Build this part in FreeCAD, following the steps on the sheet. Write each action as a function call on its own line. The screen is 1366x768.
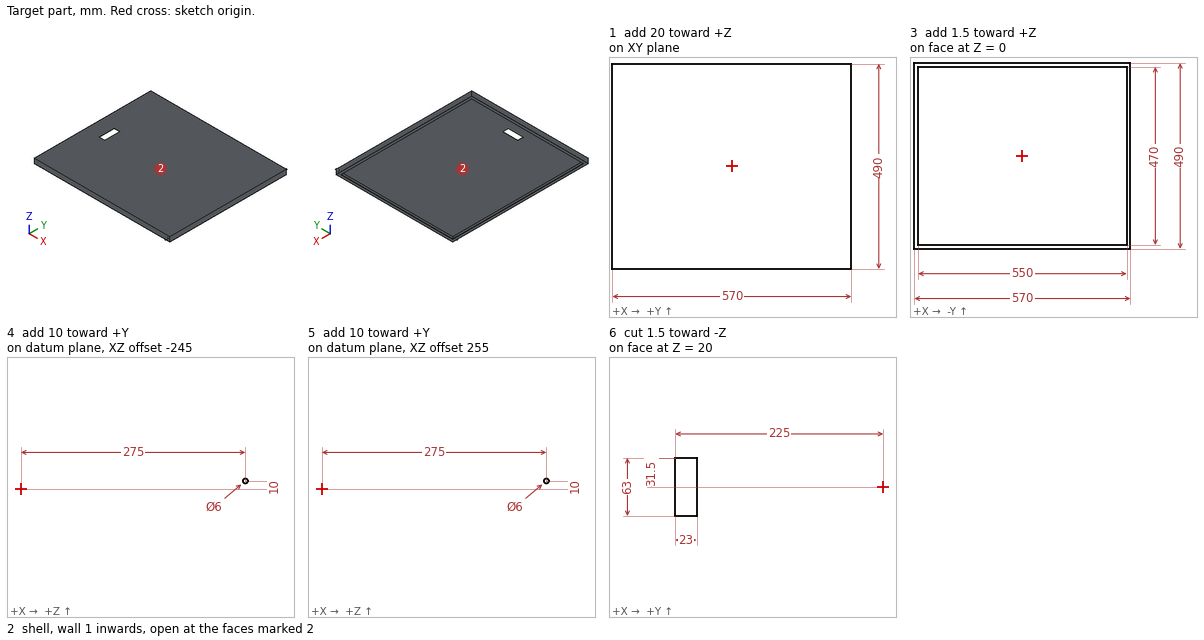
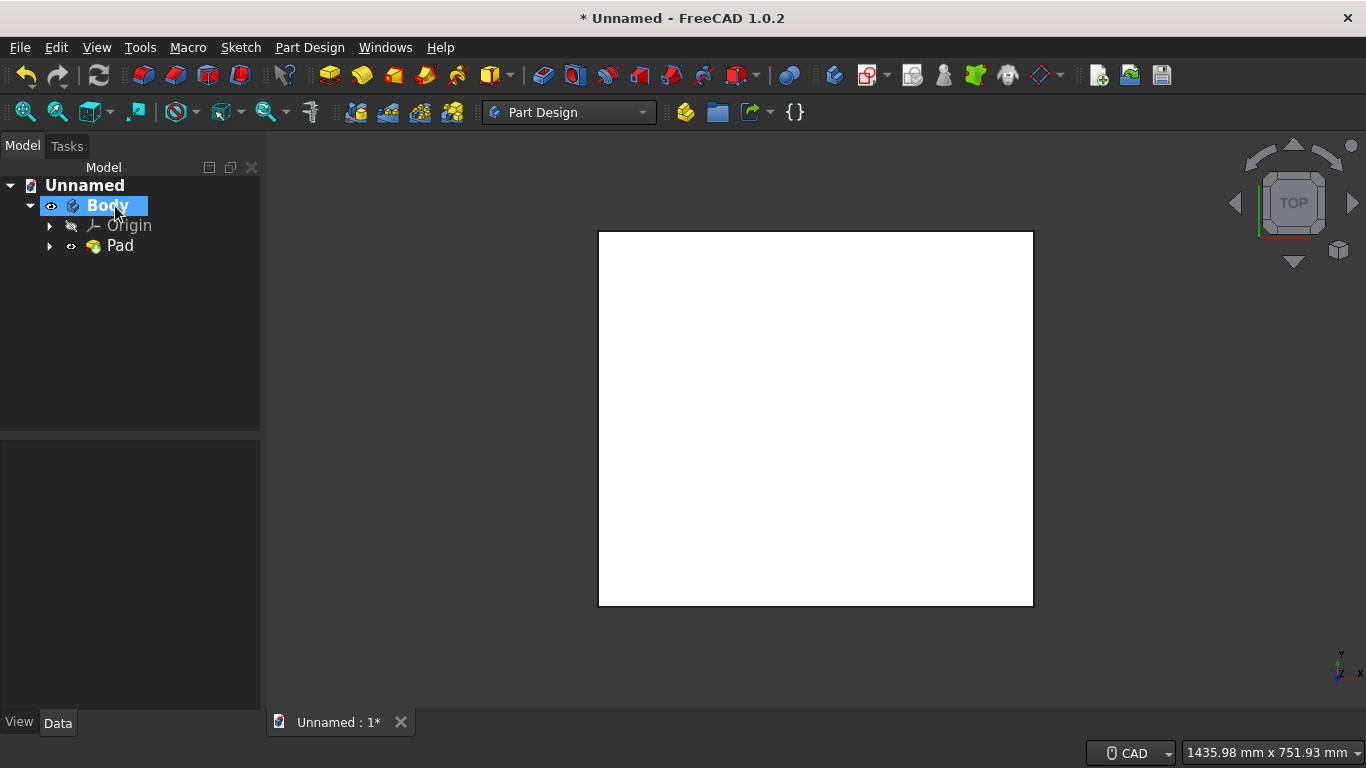
key(1)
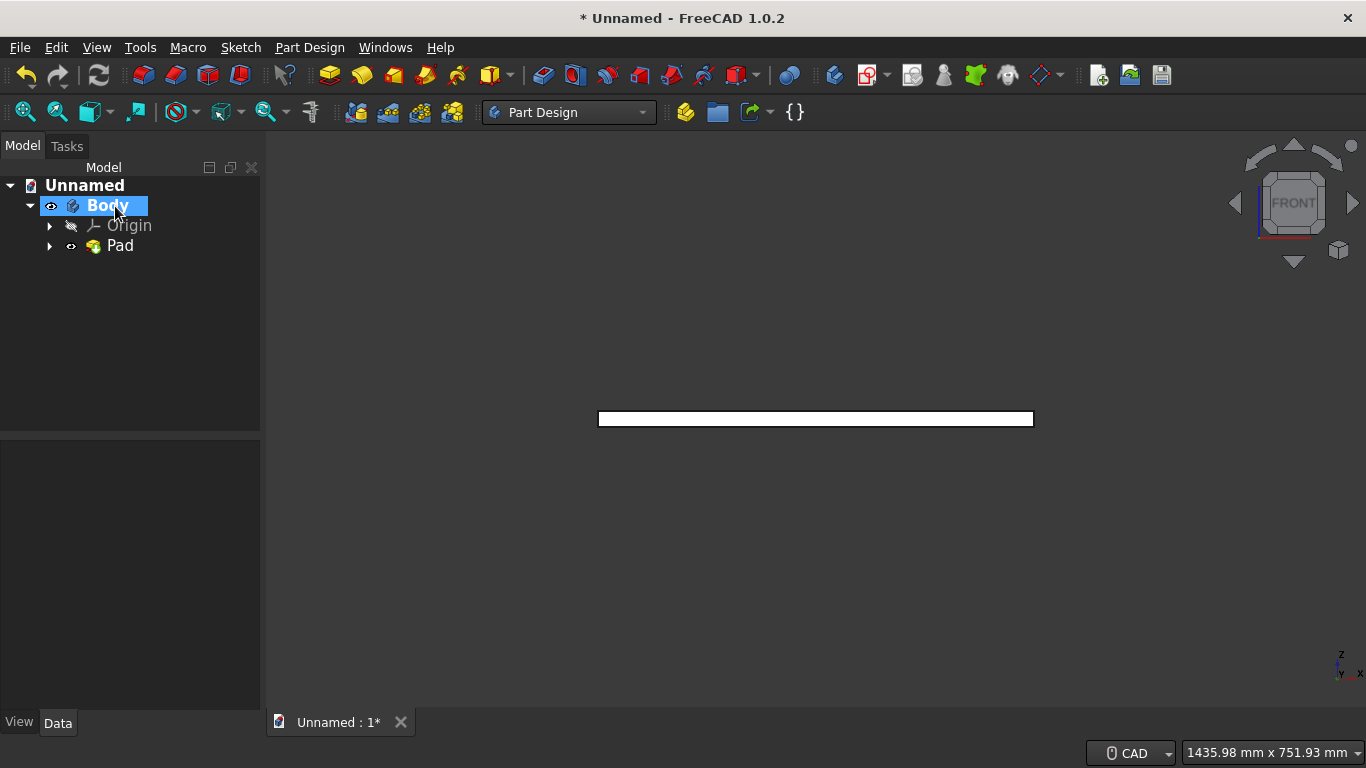
key(v)
key(f)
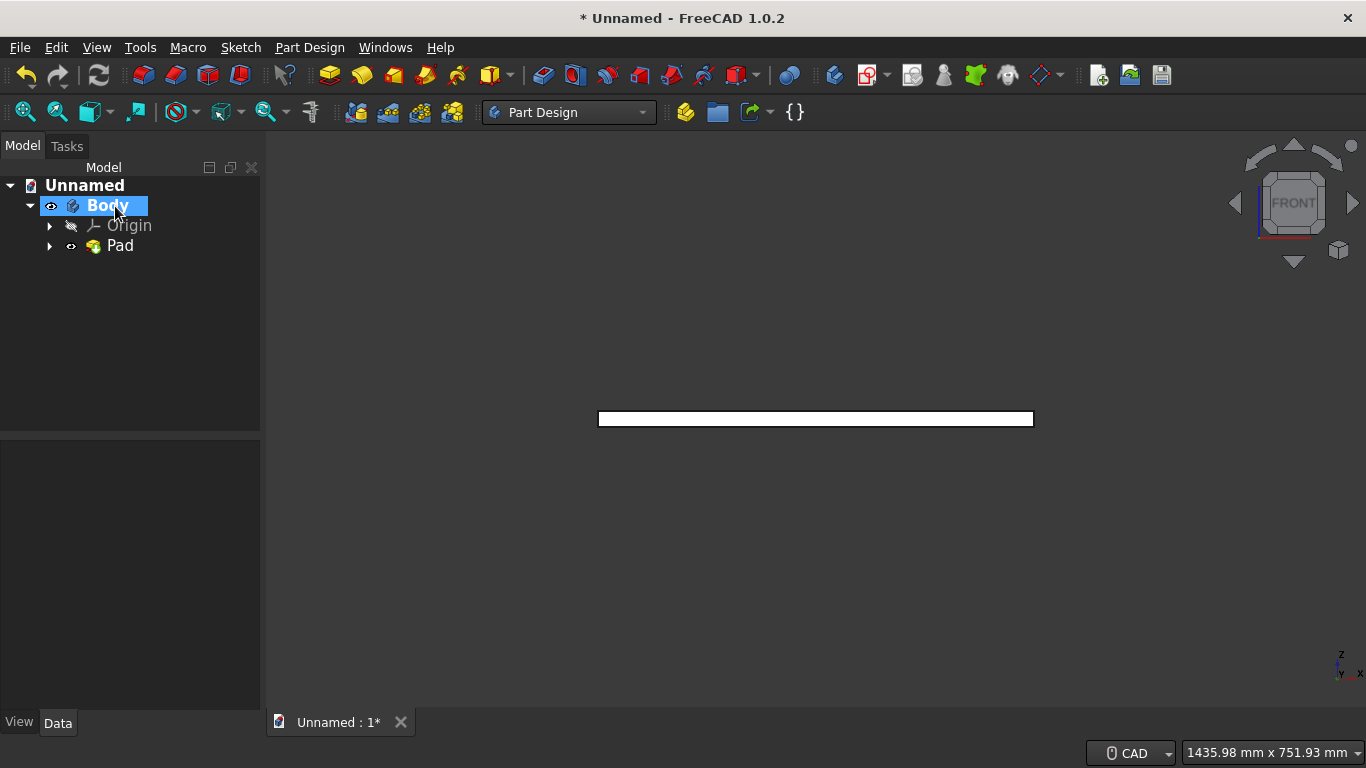
key(3)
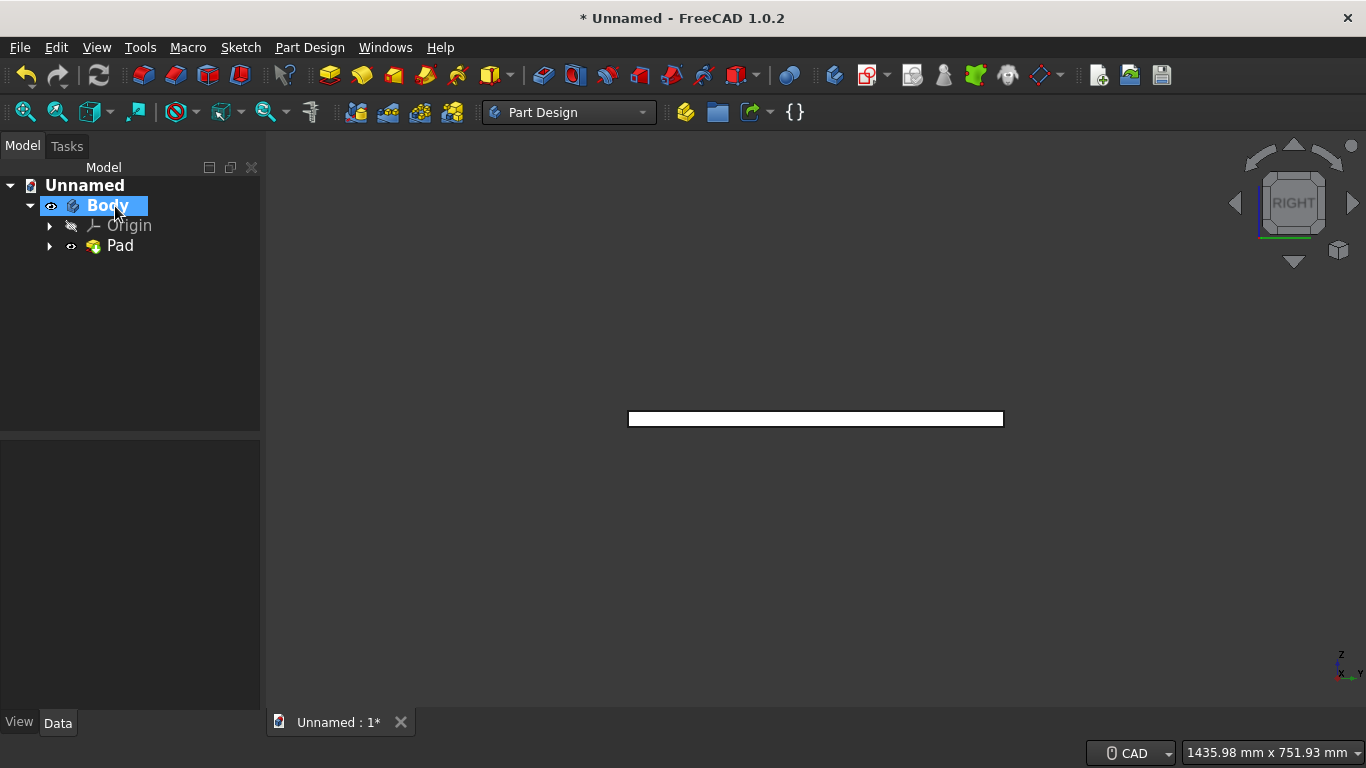
key(v)
key(f)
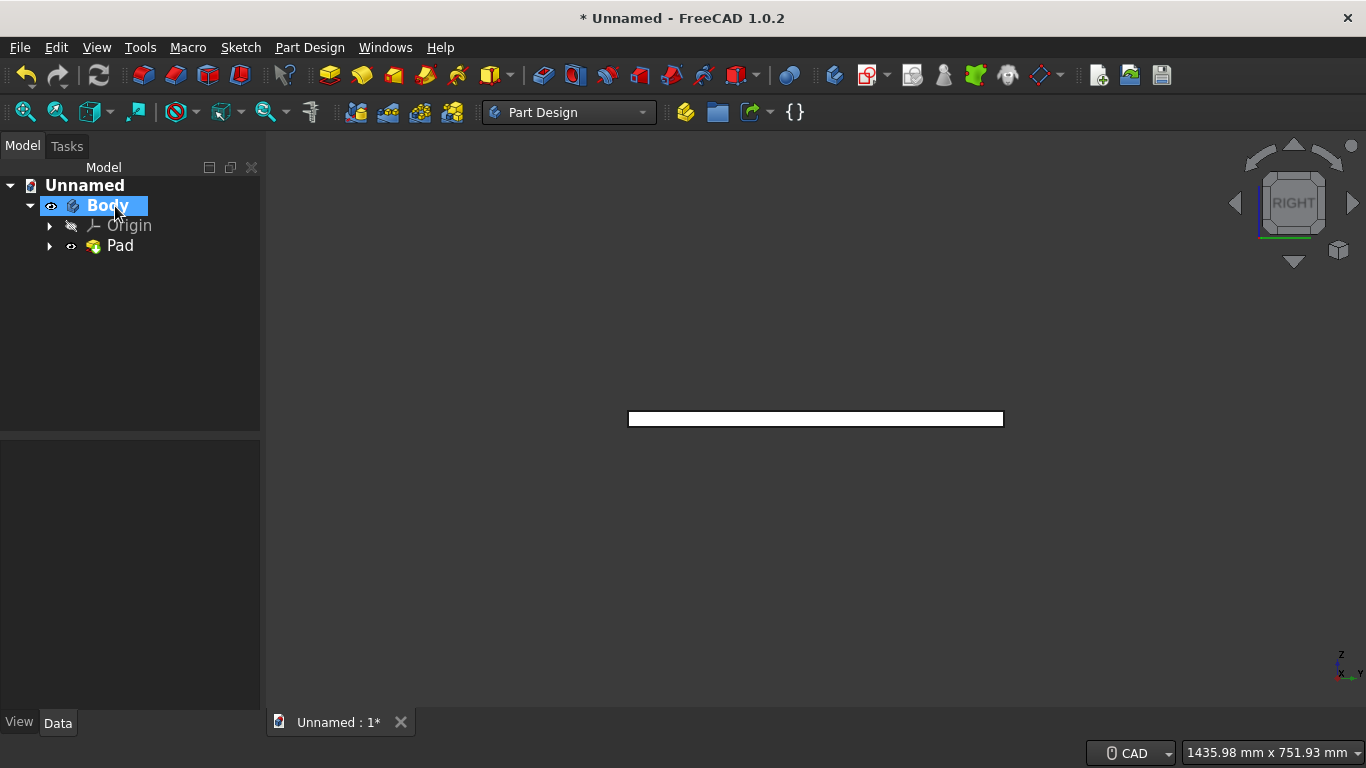
key(5)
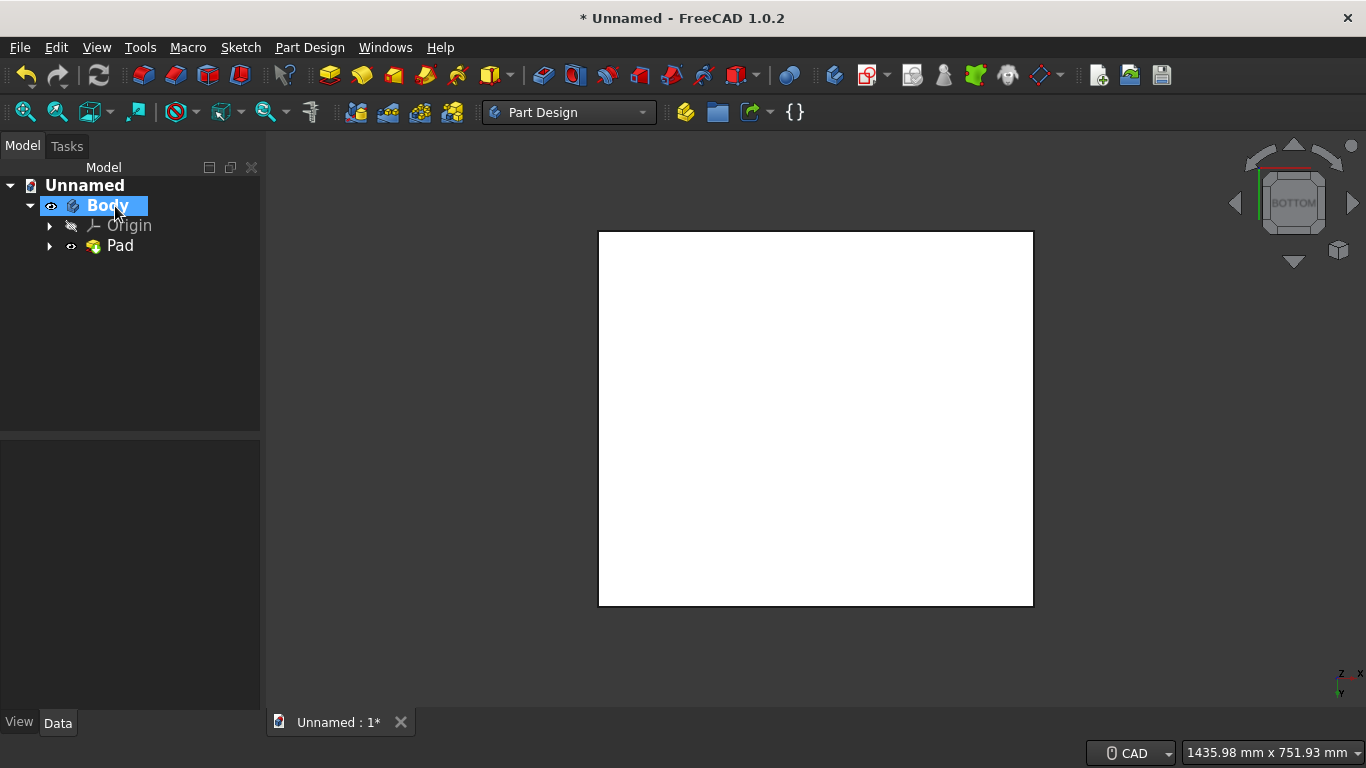
click(816, 418)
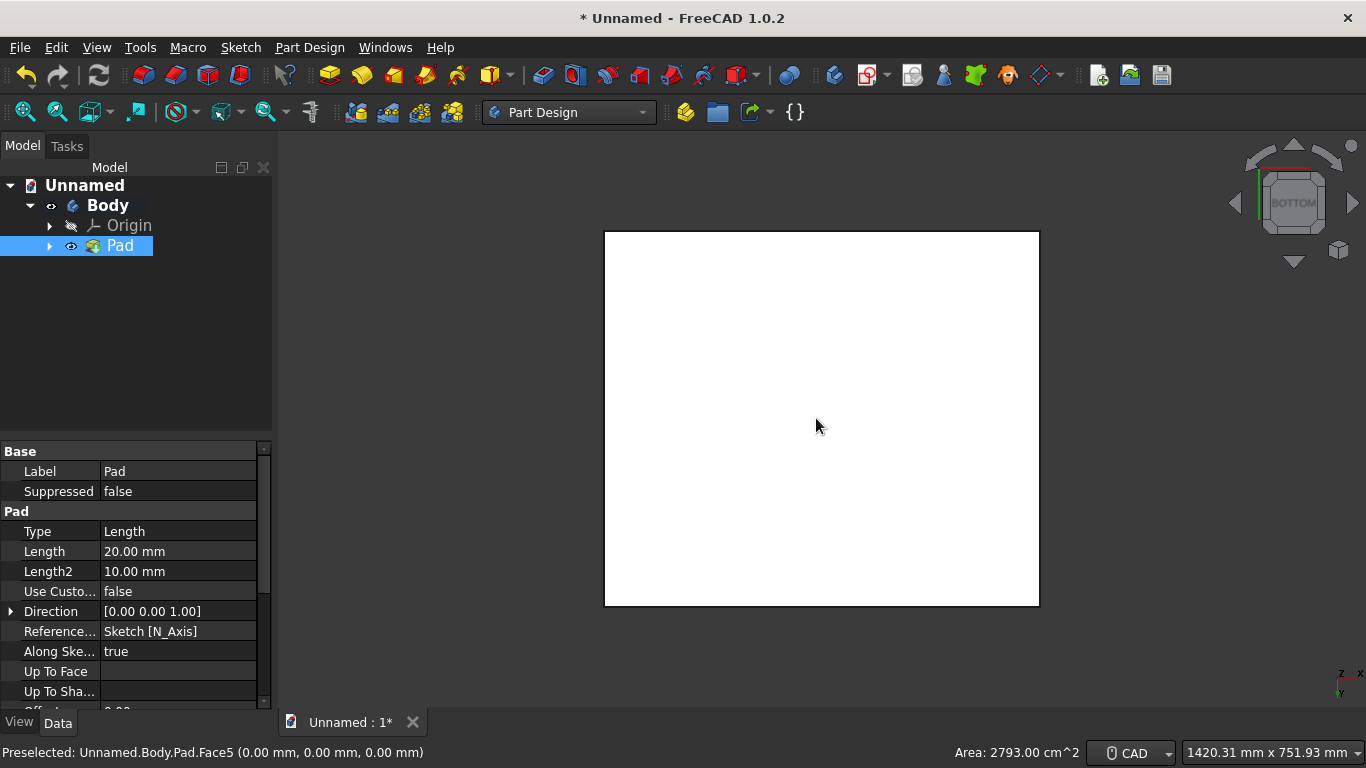
click(240, 76)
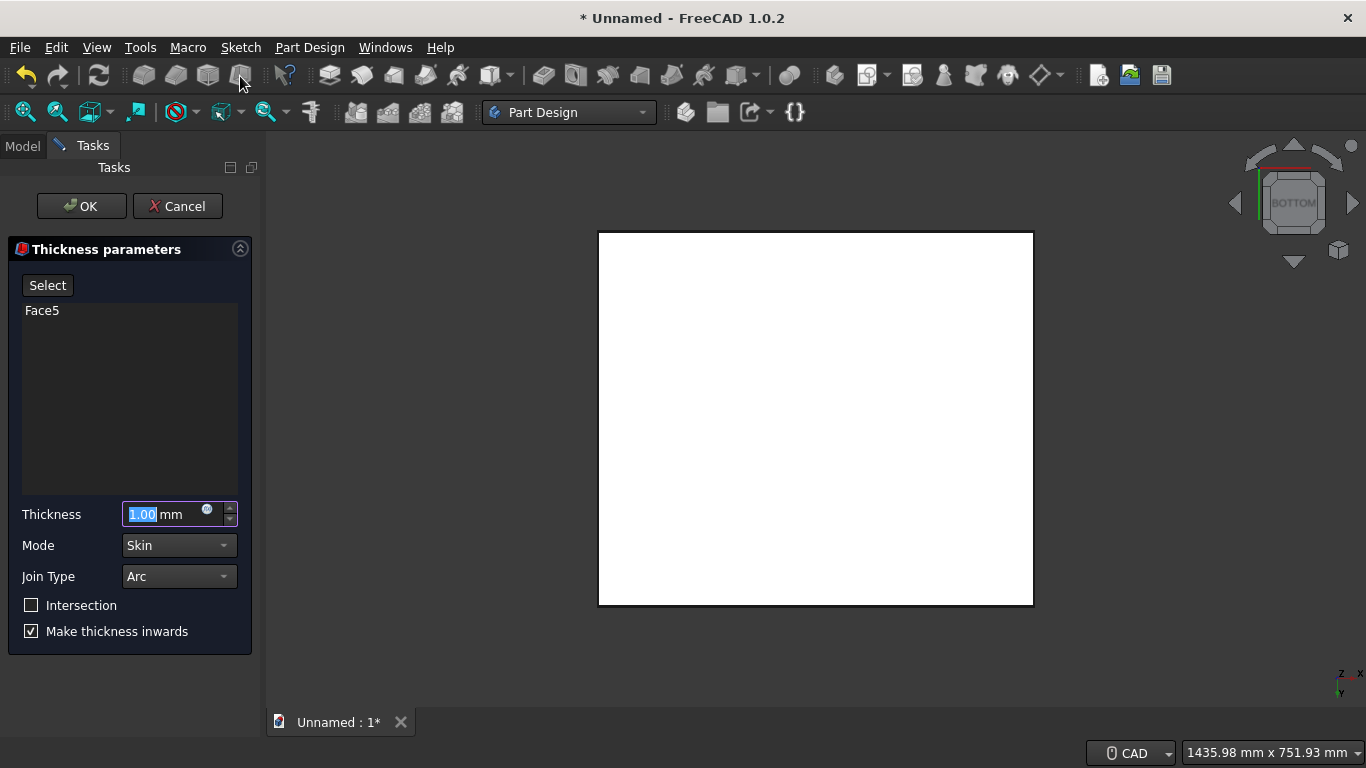
text(1)
key(Tab)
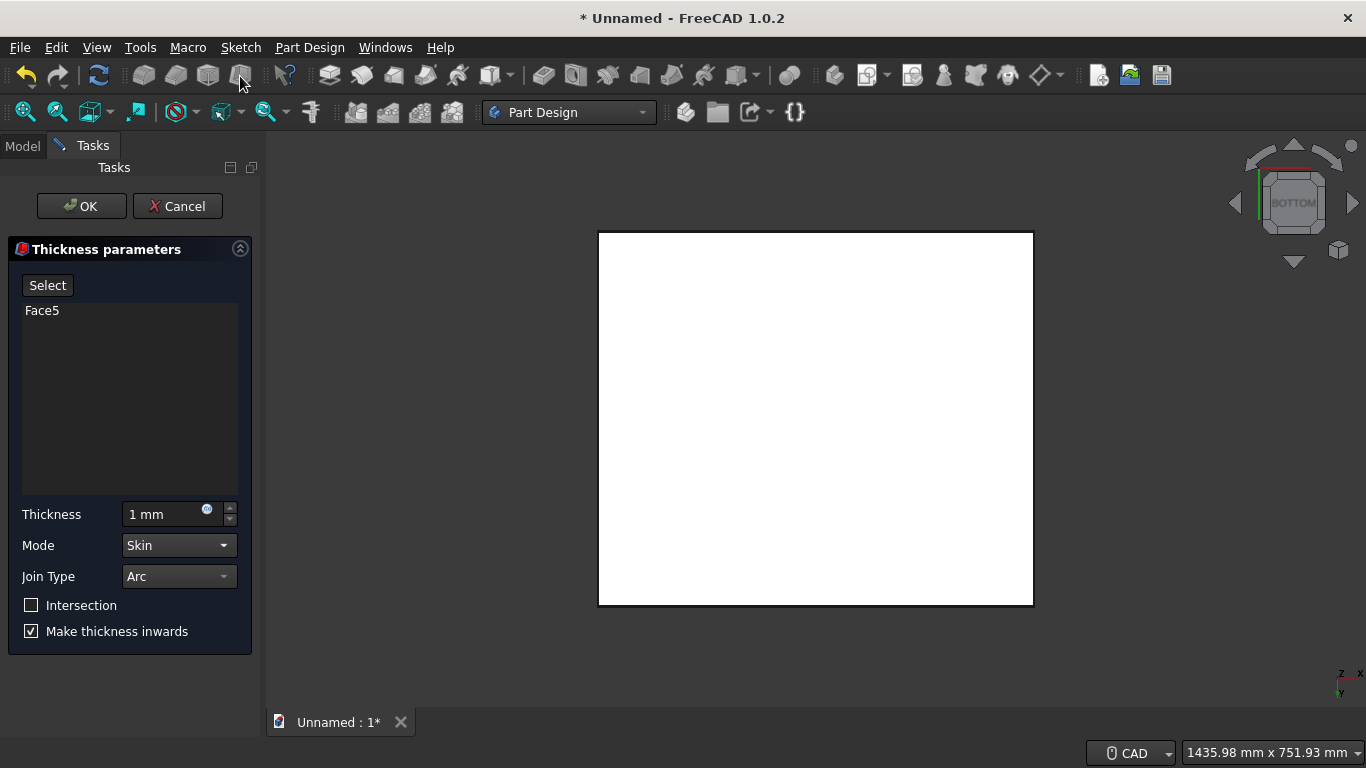
click(180, 576)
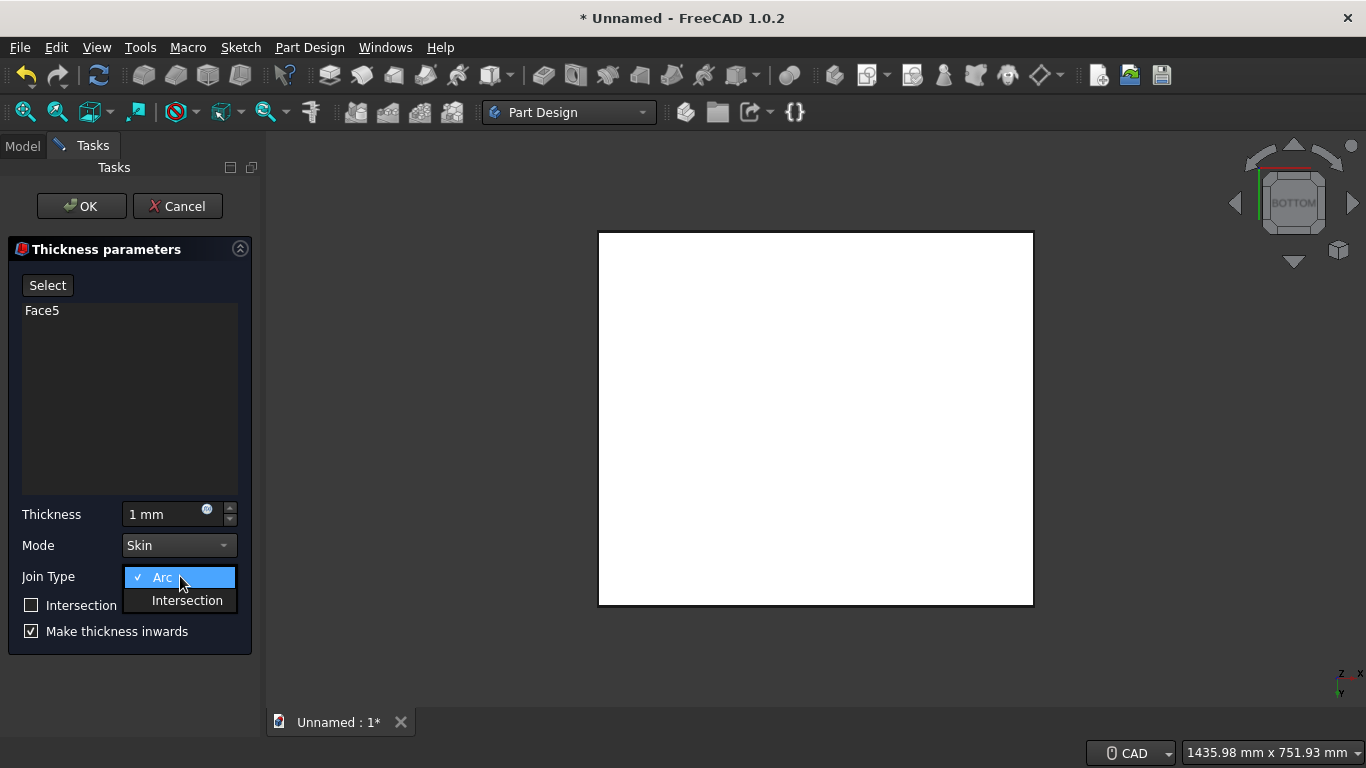
click(179, 600)